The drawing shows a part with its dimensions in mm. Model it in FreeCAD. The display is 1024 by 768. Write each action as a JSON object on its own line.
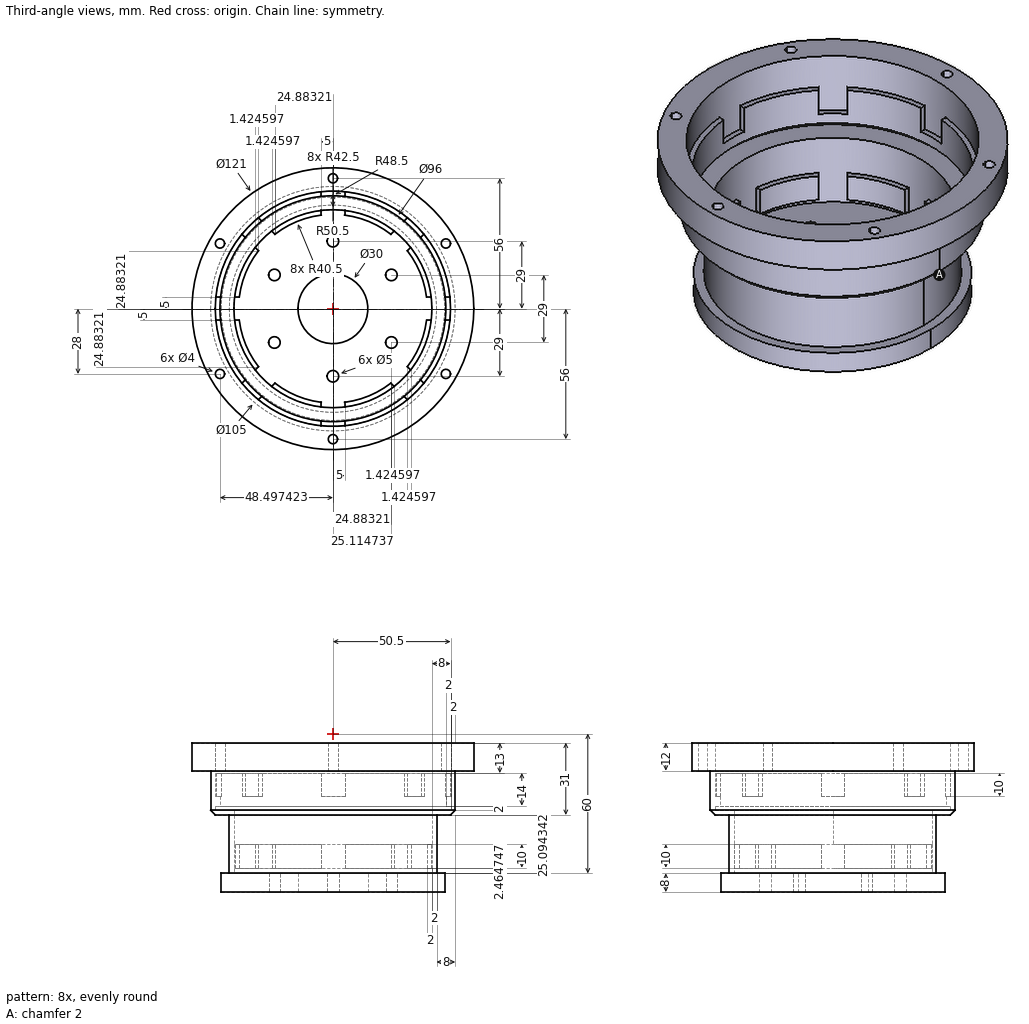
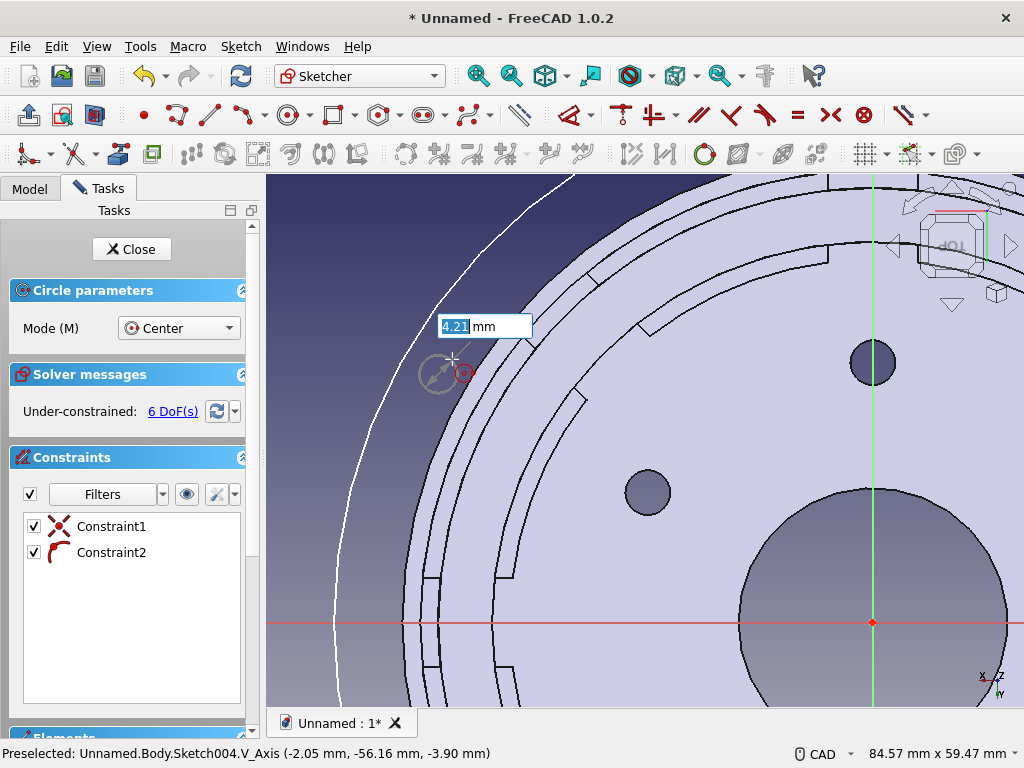
{"action": "left_click", "coordinate": [451, 359]}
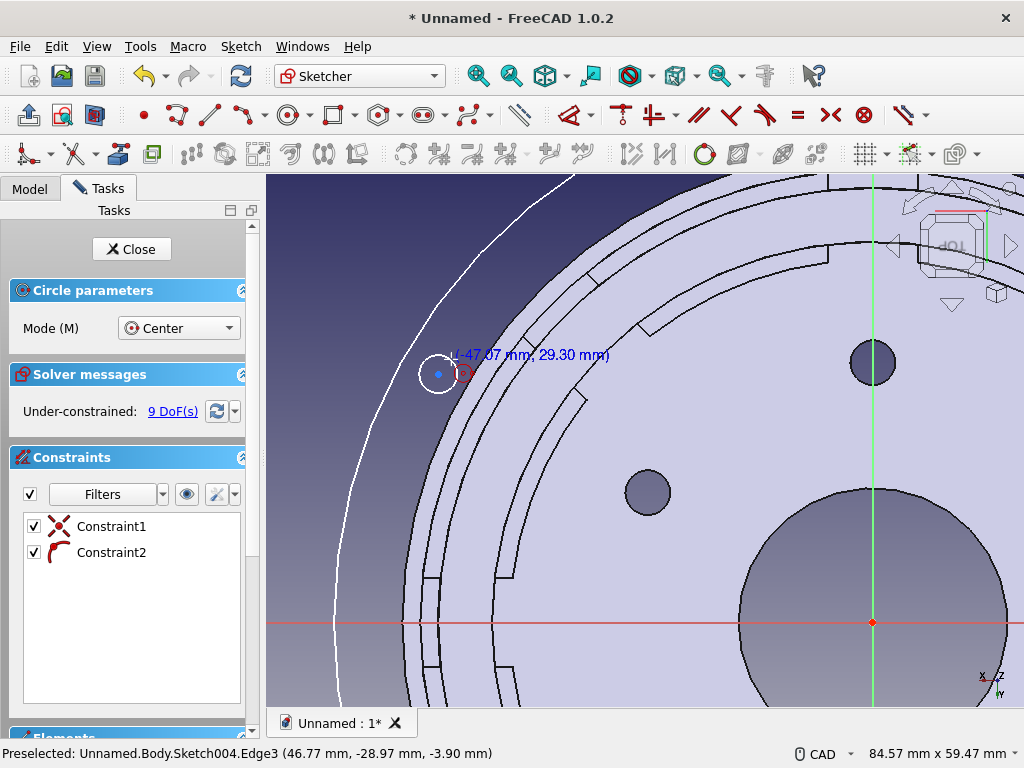
{"action": "scroll", "coordinate": [449, 362], "scroll_direction": "down", "scroll_amount": 6}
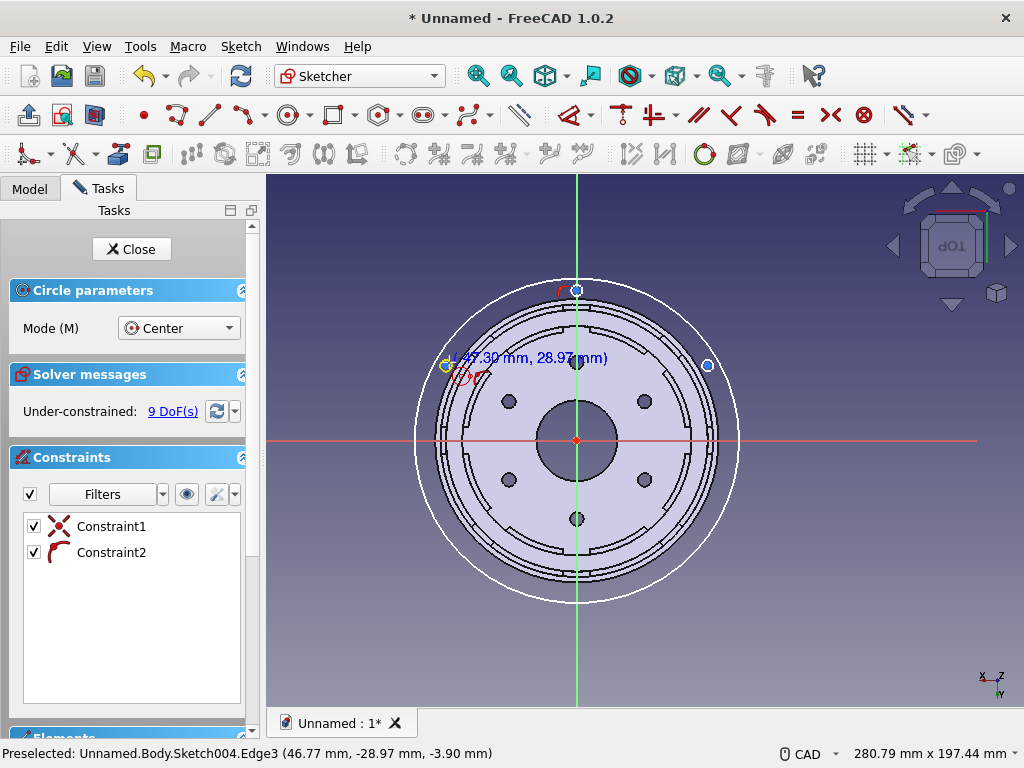
{"action": "scroll", "coordinate": [708, 516], "scroll_direction": "up", "scroll_amount": 8}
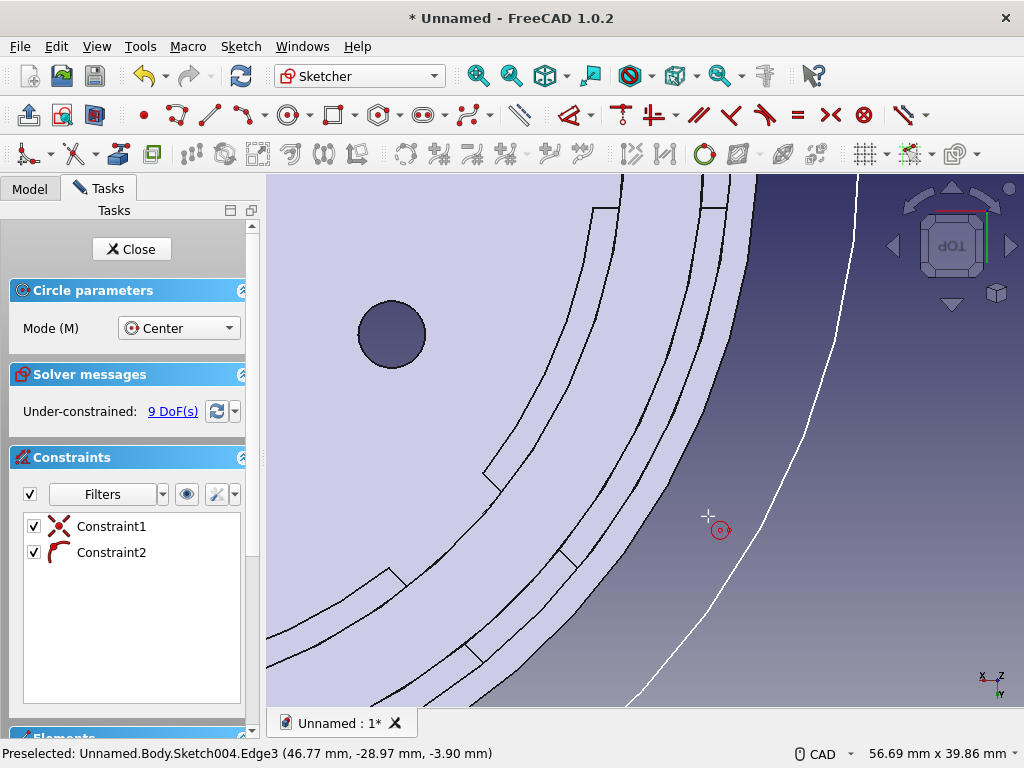
{"action": "scroll", "coordinate": [708, 516], "scroll_direction": "down", "scroll_amount": 8}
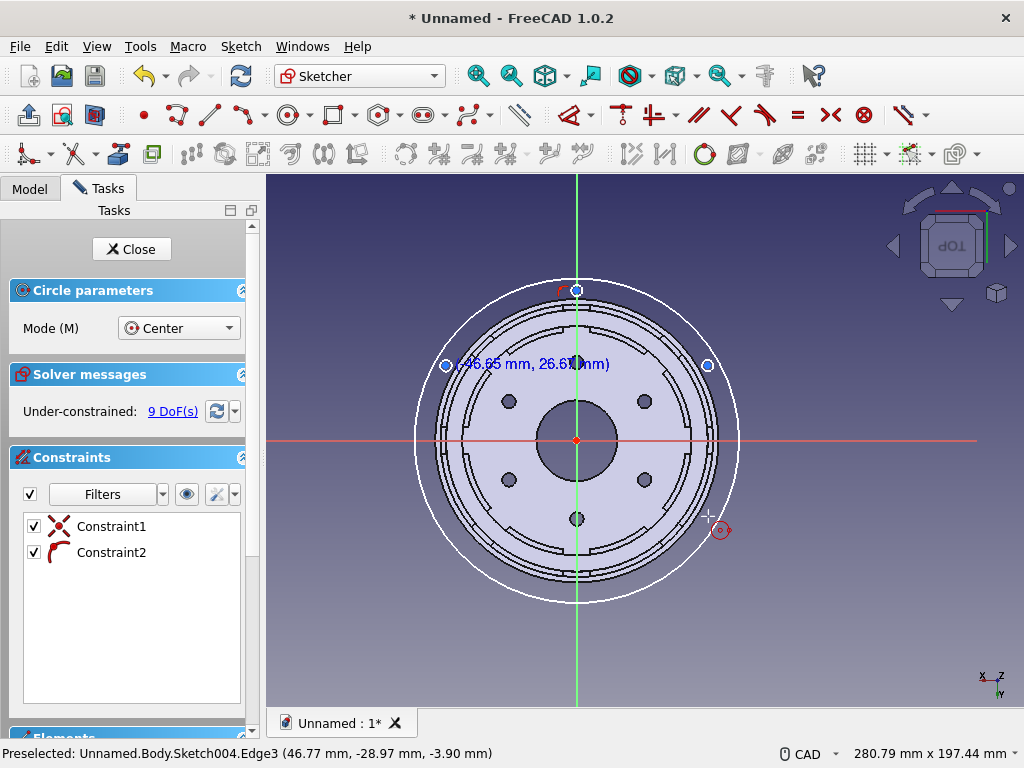
{"action": "scroll", "coordinate": [708, 516], "scroll_direction": "up", "scroll_amount": 2}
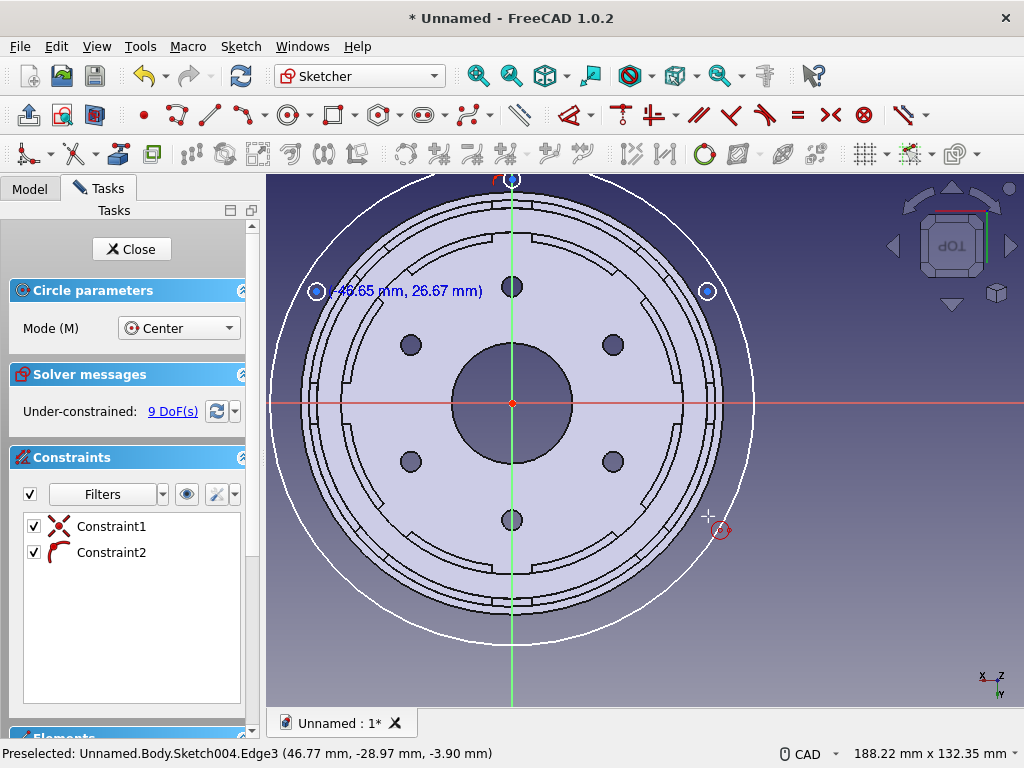
{"action": "left_click", "coordinate": [707, 516]}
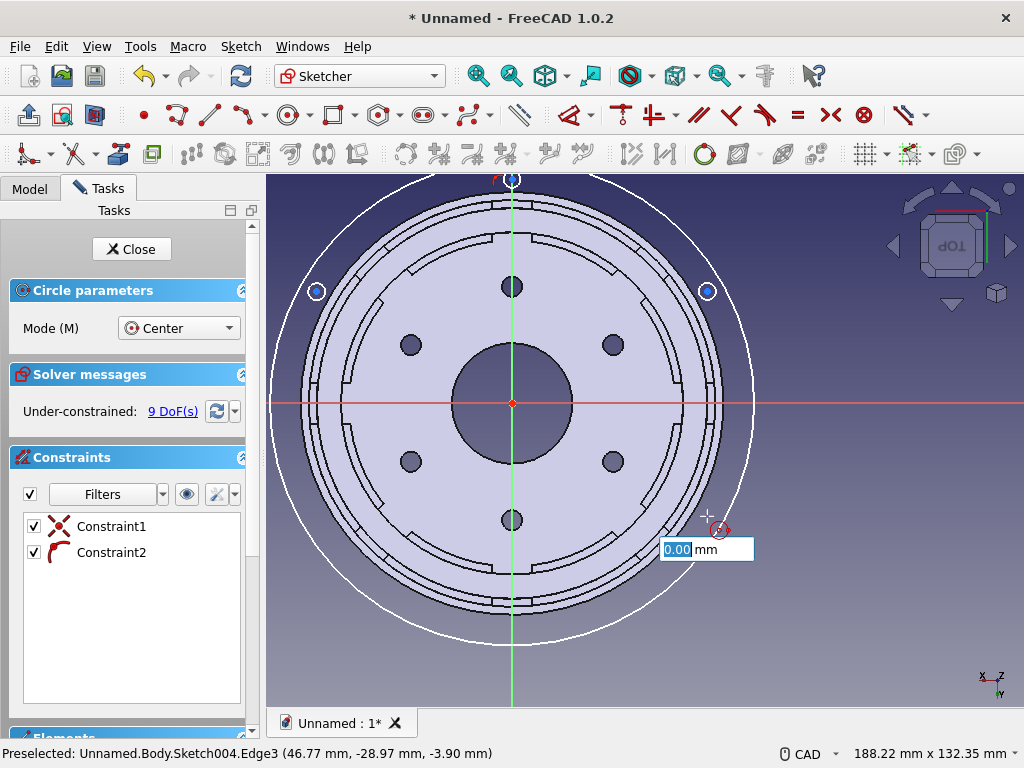
{"action": "scroll", "coordinate": [713, 510], "scroll_direction": "up", "scroll_amount": 4}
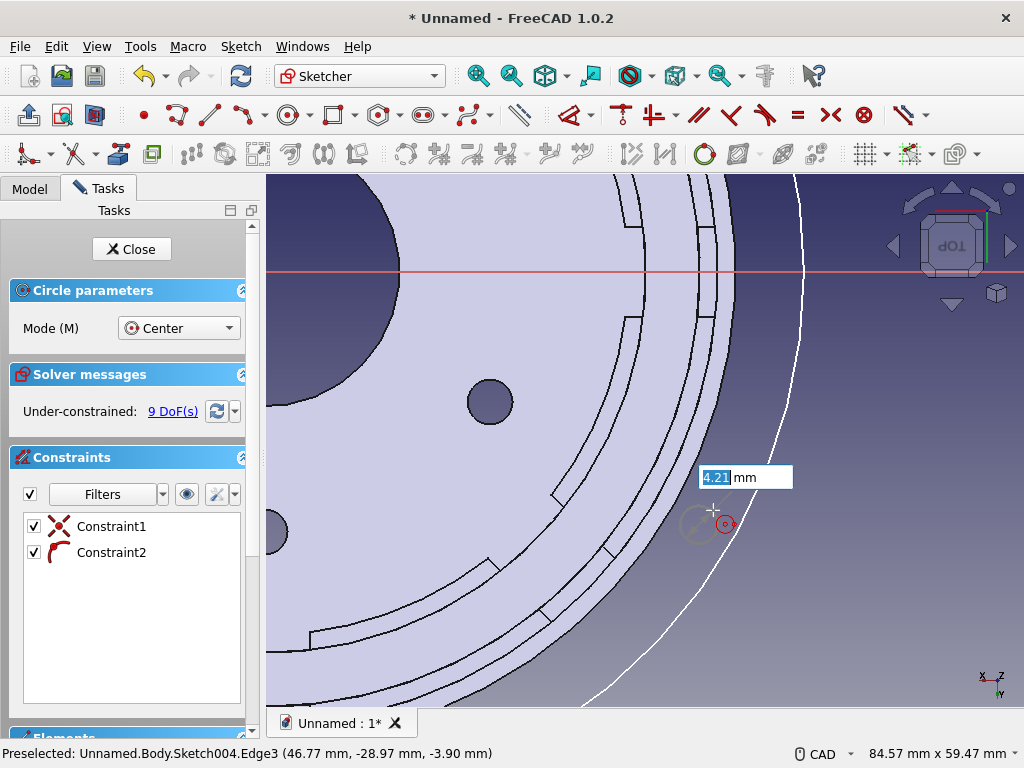
{"action": "left_click", "coordinate": [712, 510]}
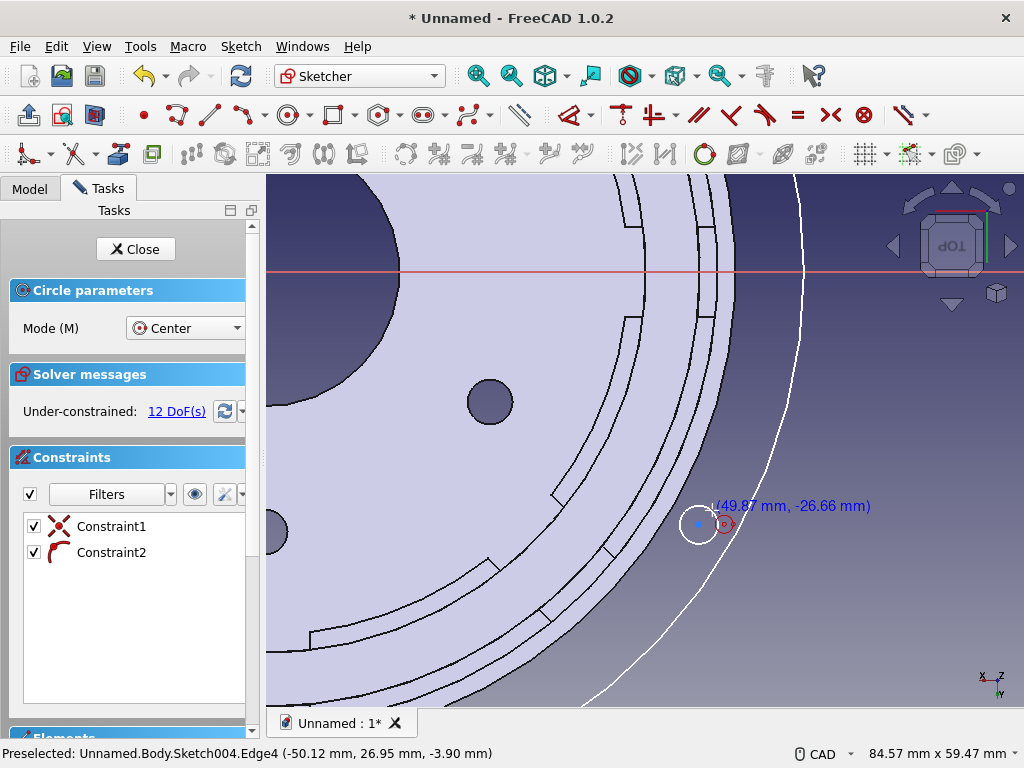
{"action": "scroll", "coordinate": [711, 513], "scroll_direction": "down", "scroll_amount": 6}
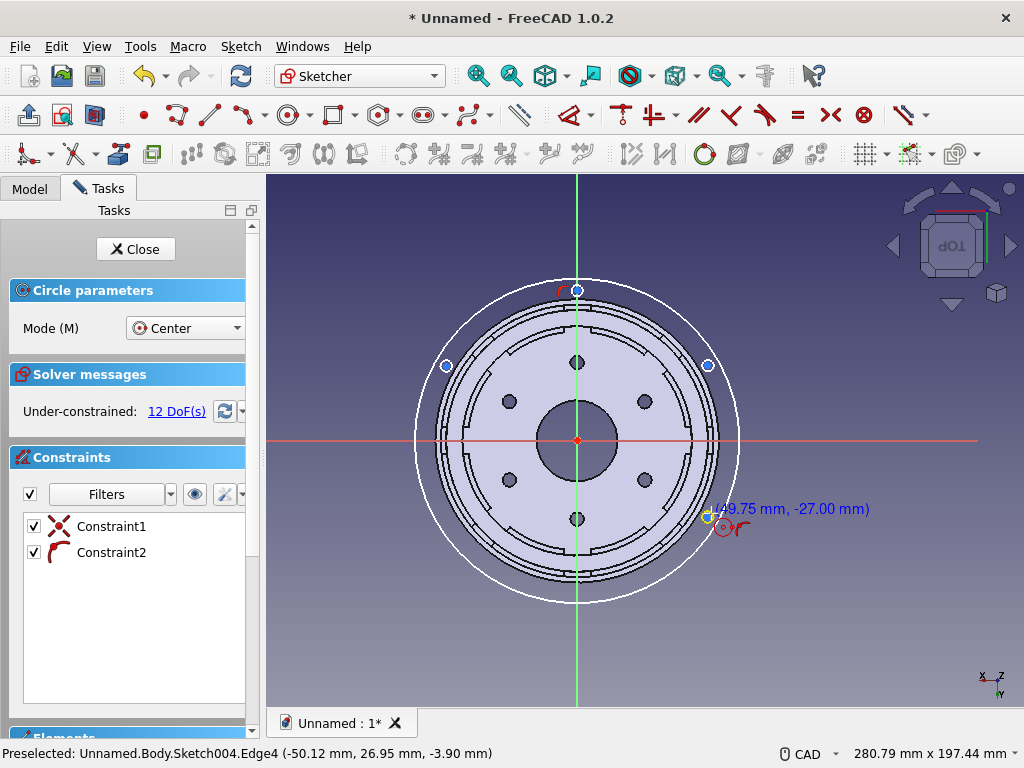
{"action": "left_click", "coordinate": [577, 441]}
{"action": "left_click", "coordinate": [677, 341]}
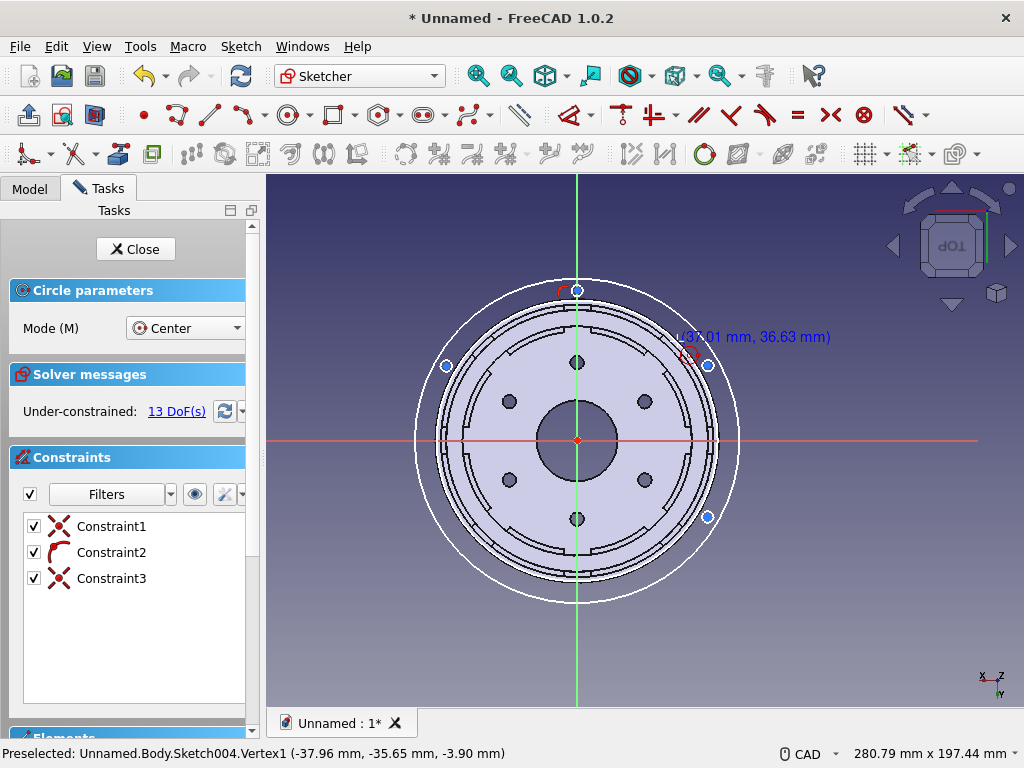
{"action": "scroll", "coordinate": [446, 516], "scroll_direction": "up", "scroll_amount": 8}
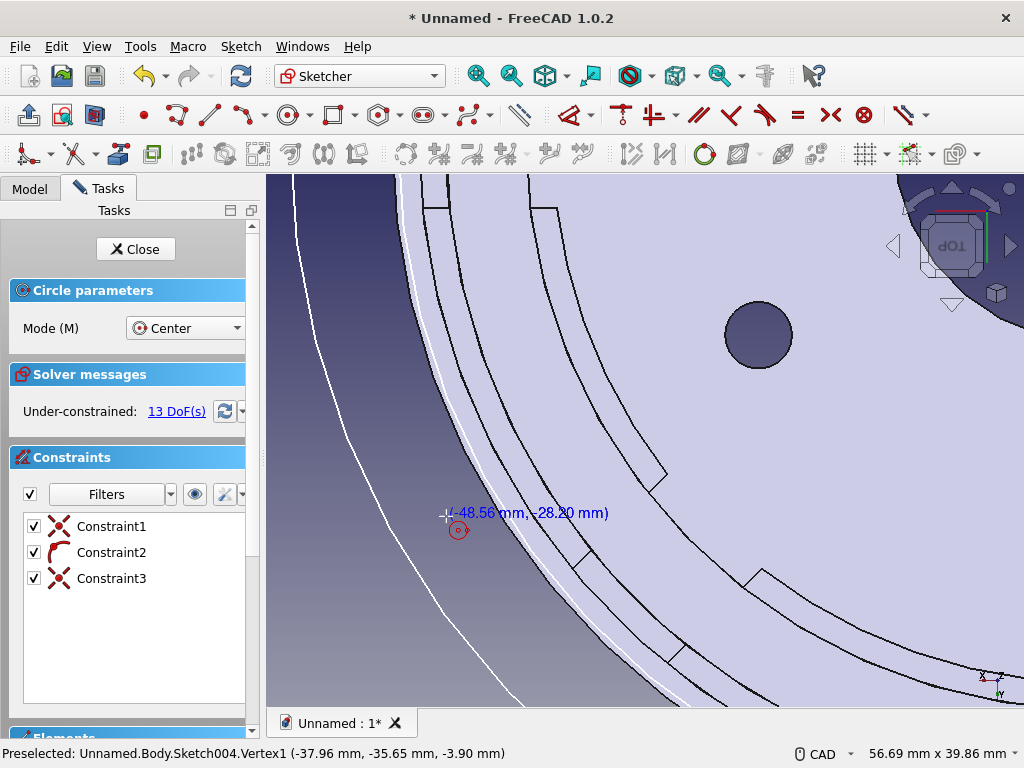
{"action": "scroll", "coordinate": [445, 516], "scroll_direction": "down", "scroll_amount": 8}